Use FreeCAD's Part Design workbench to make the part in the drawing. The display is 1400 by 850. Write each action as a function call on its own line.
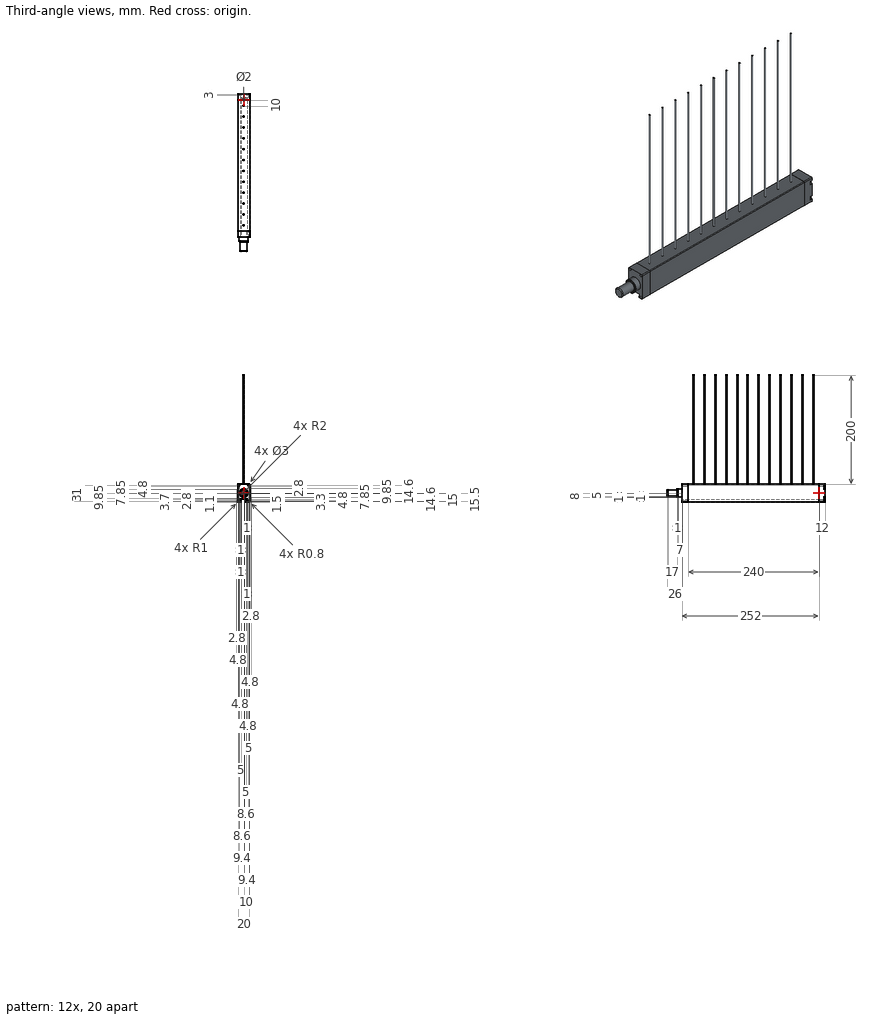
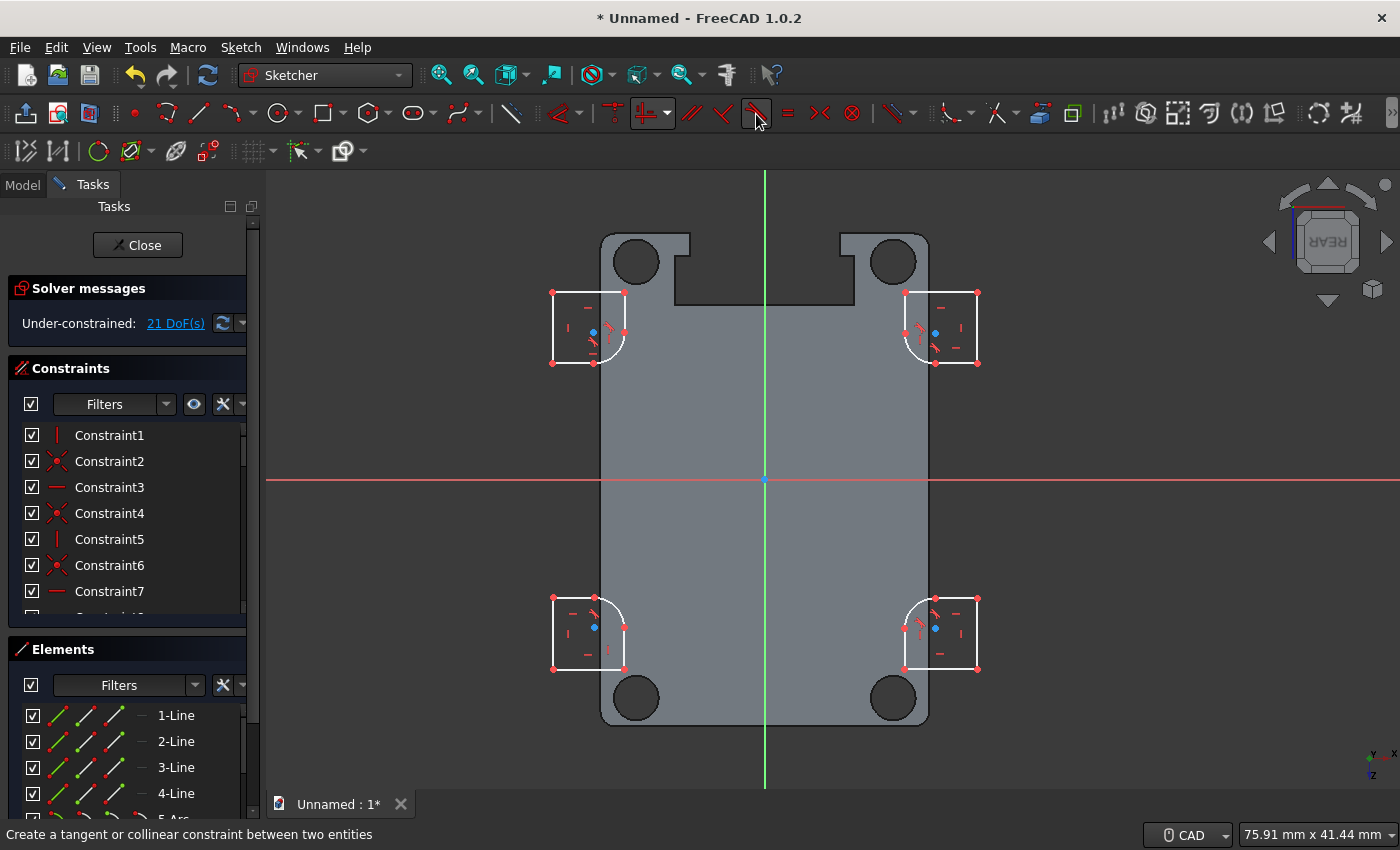
click(624, 657)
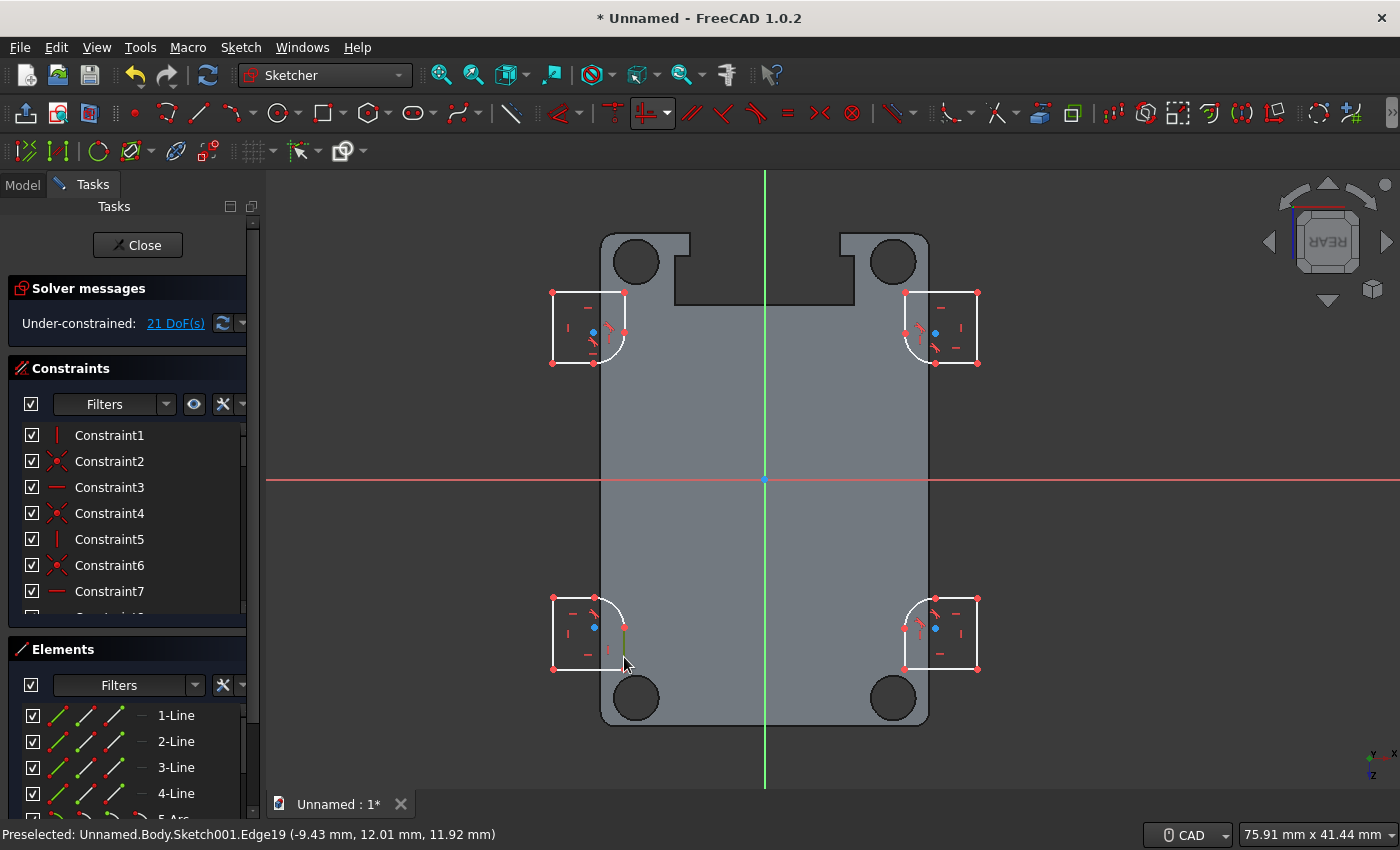
click(621, 614)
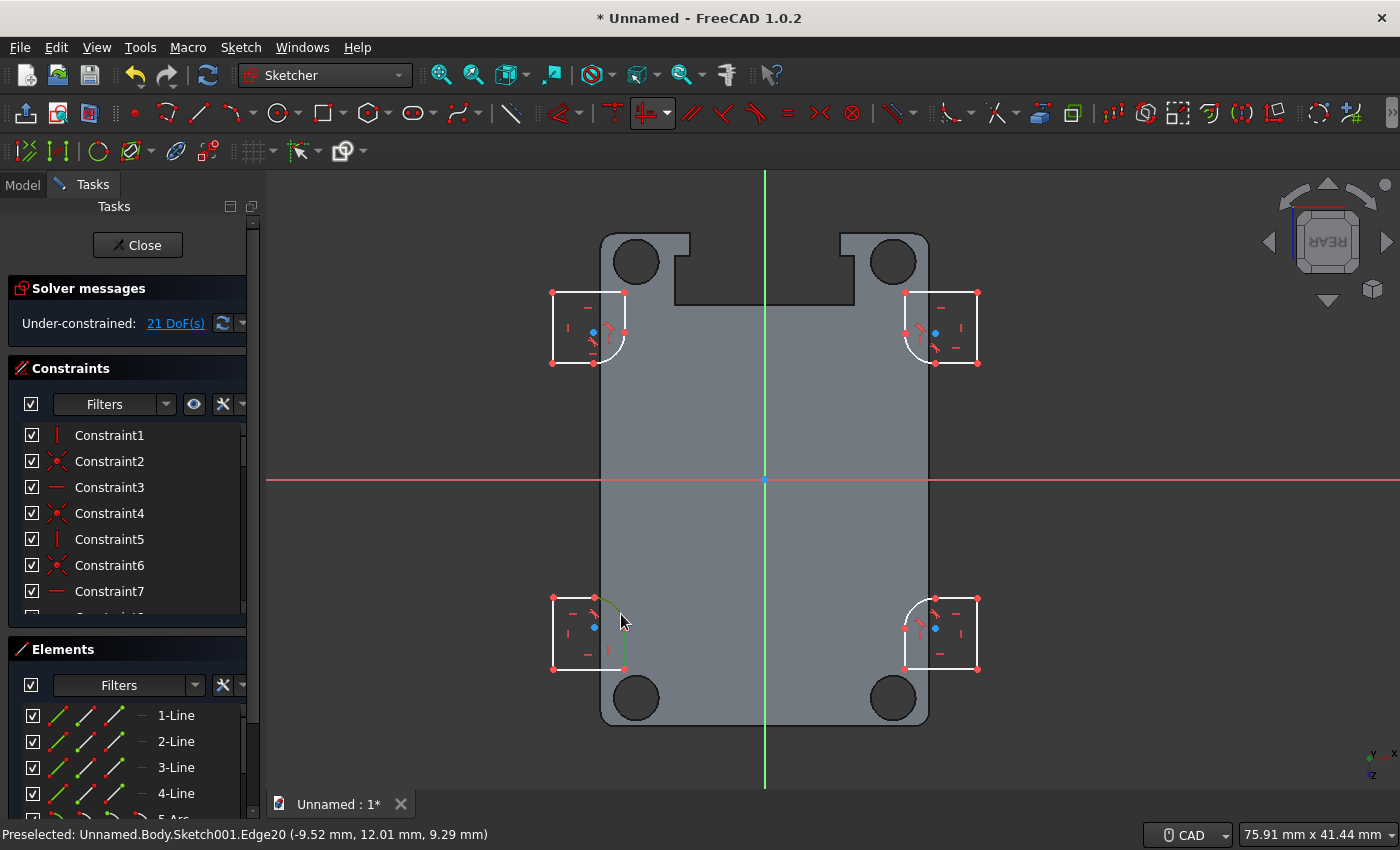
click(756, 114)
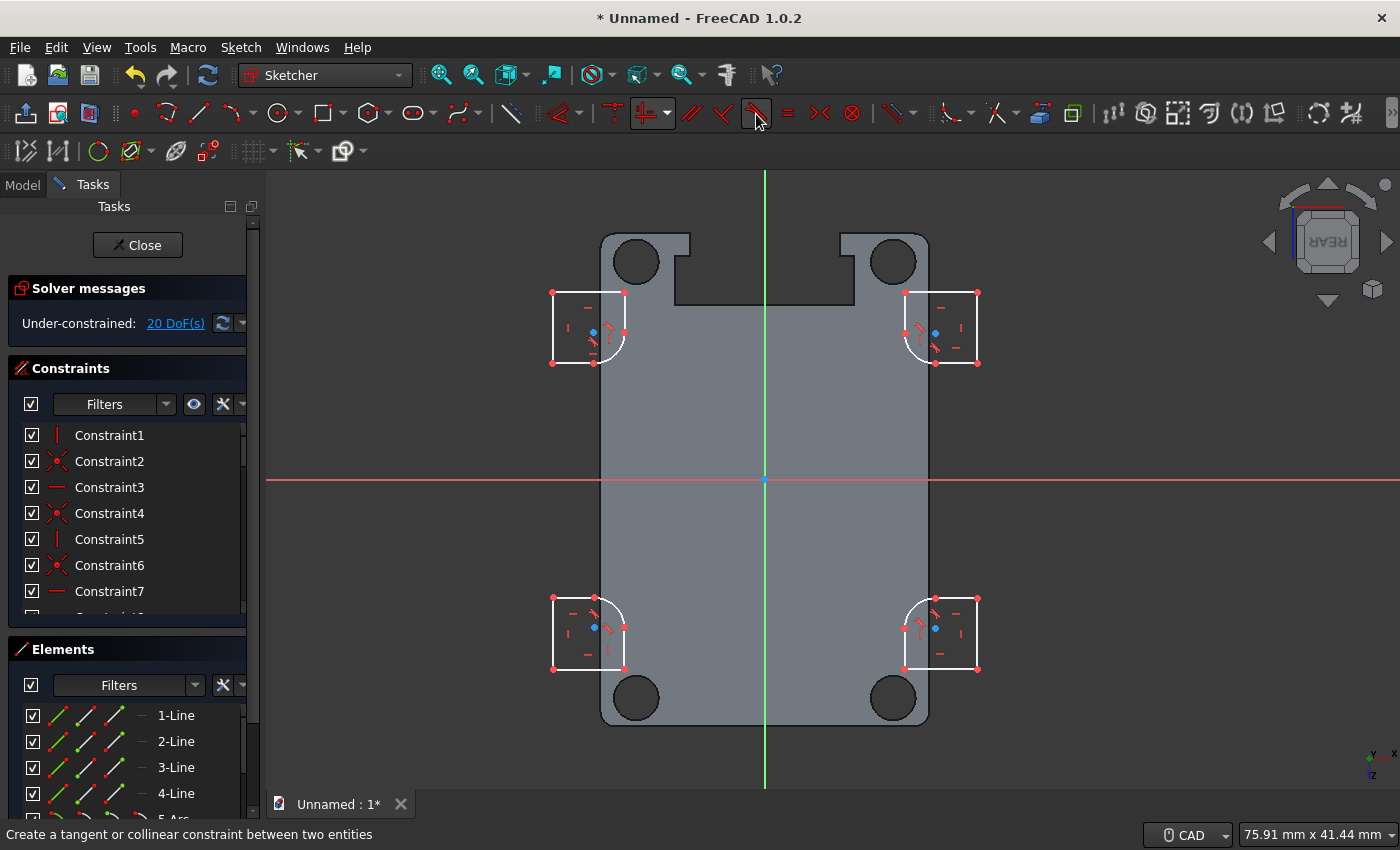
click(608, 360)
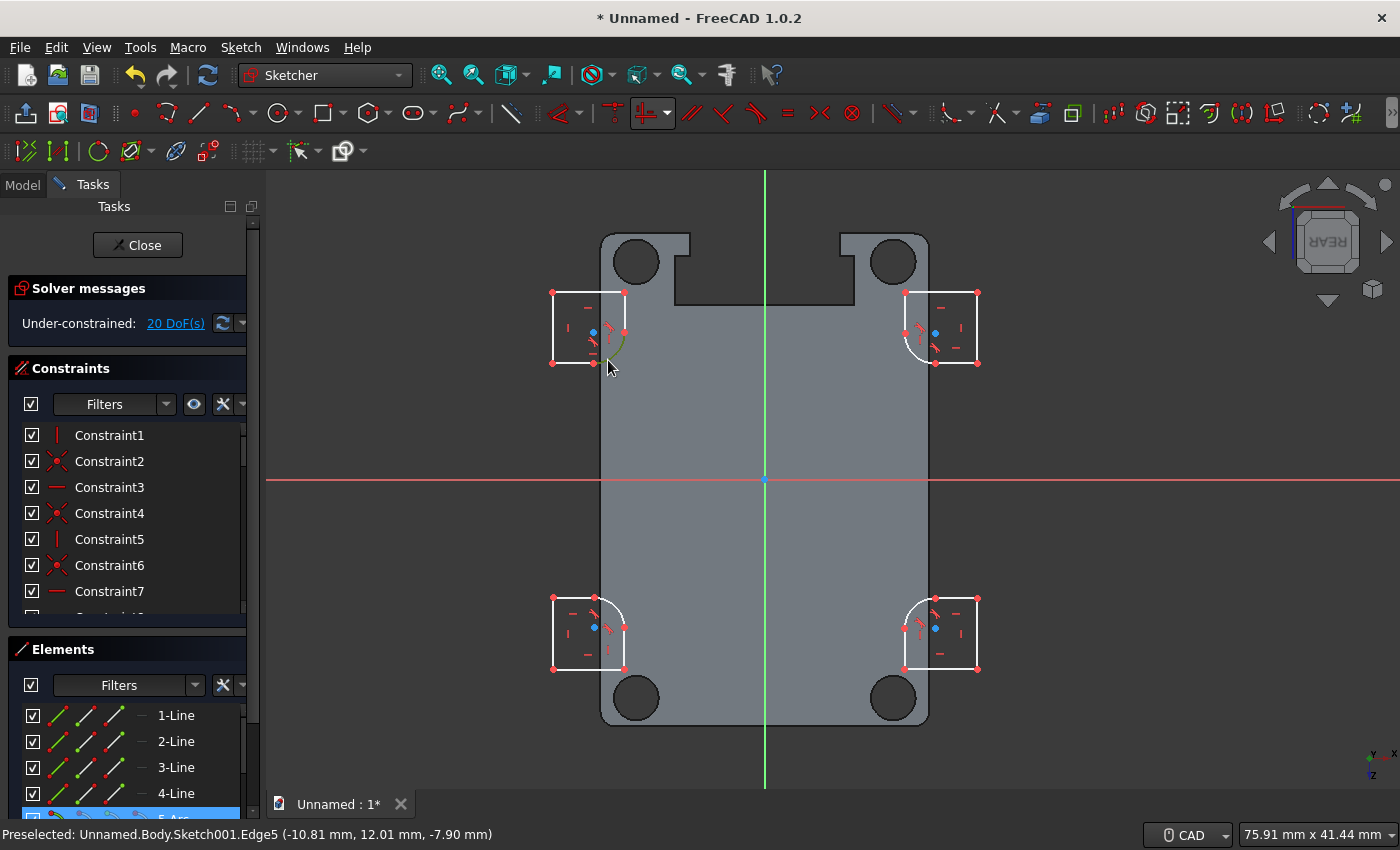
click(908, 347)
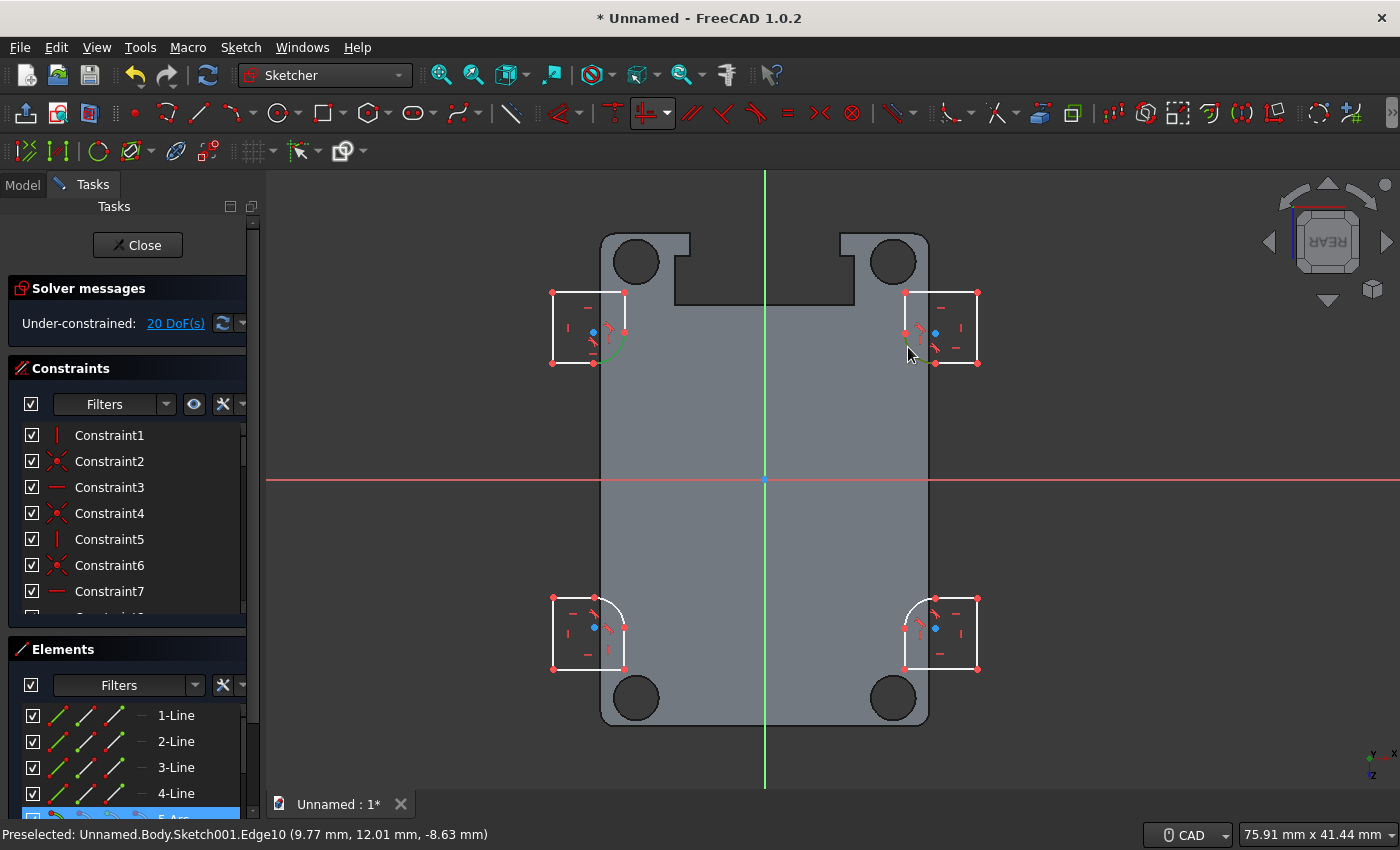
click(921, 602)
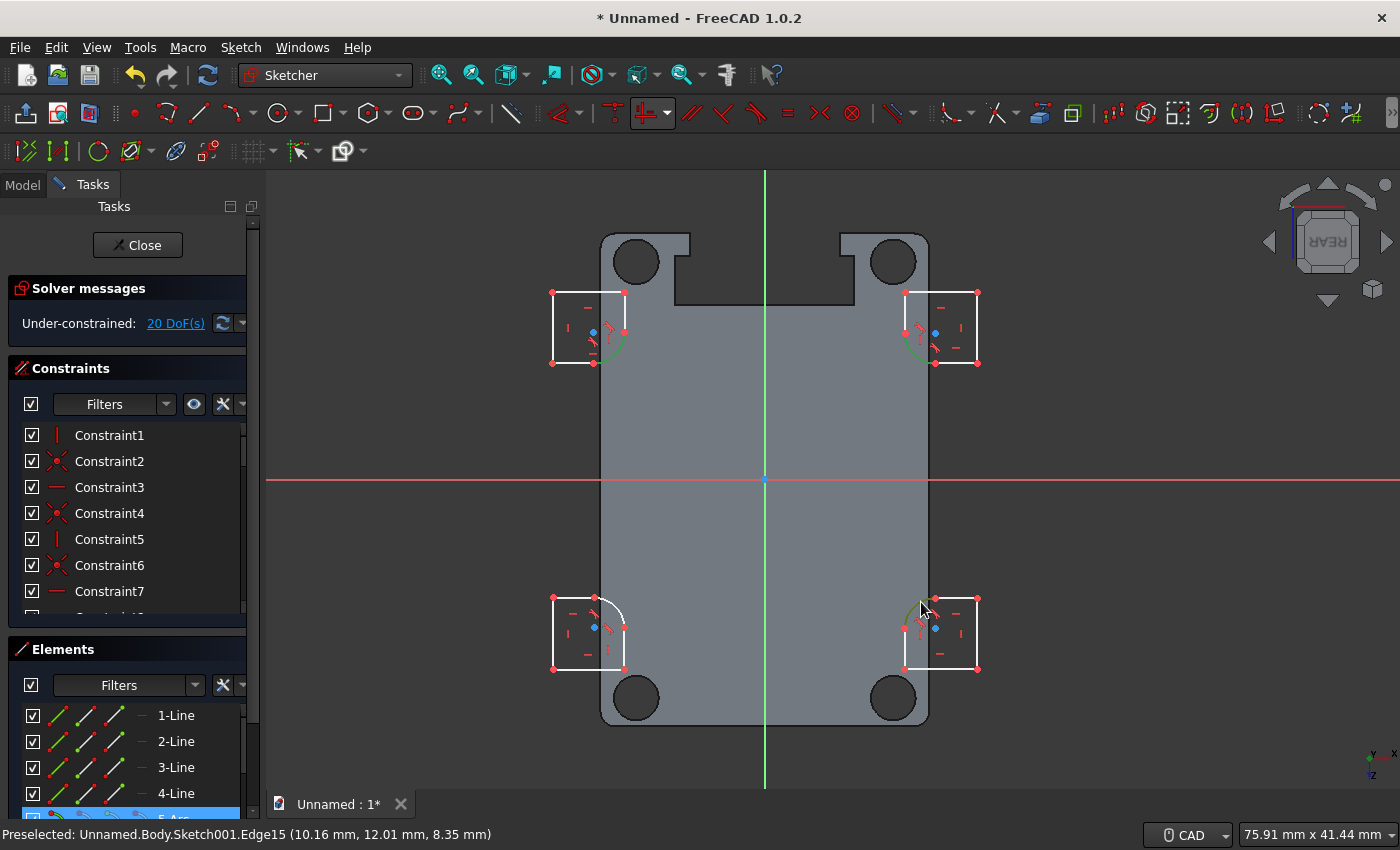
click(621, 614)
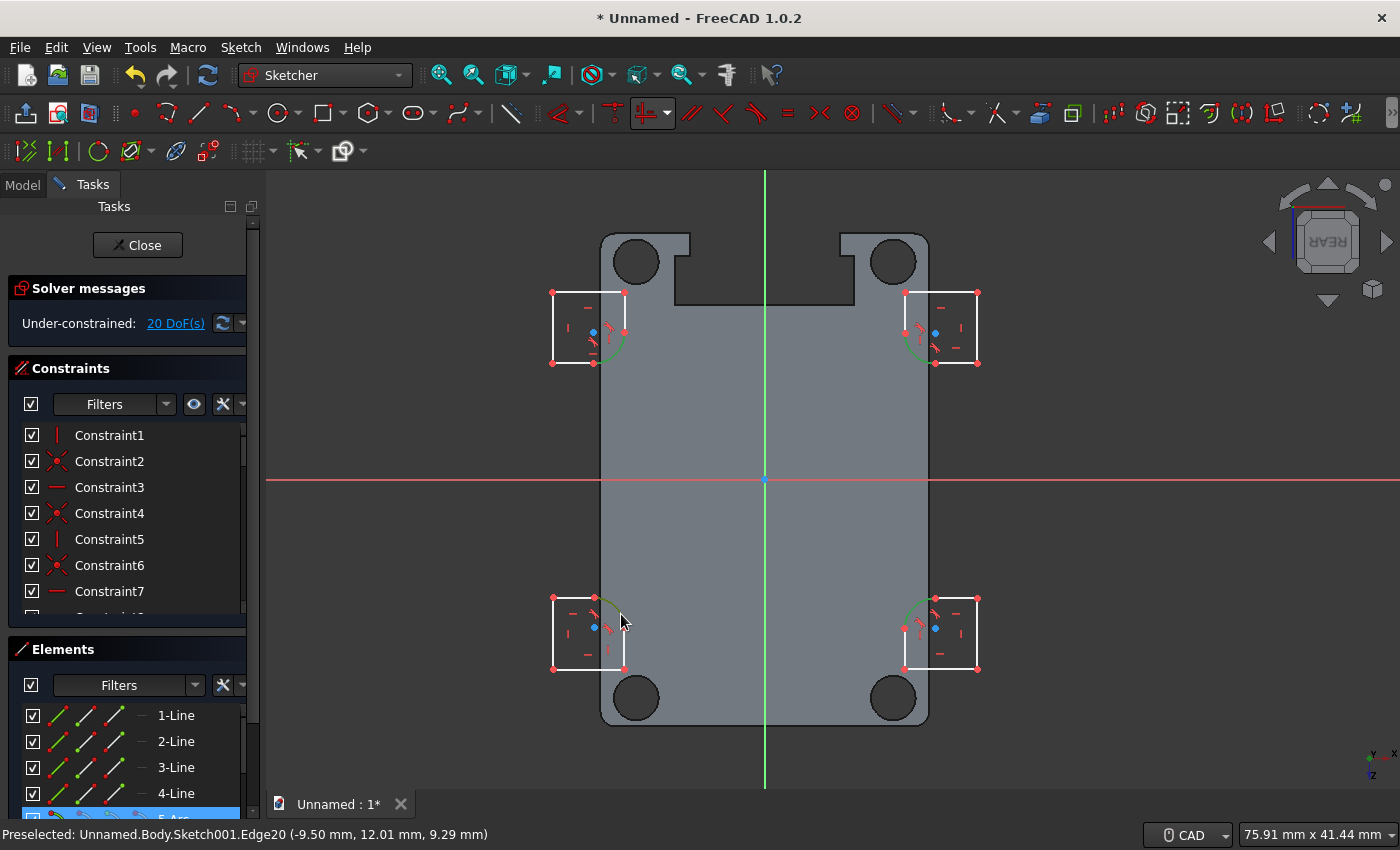
click(788, 114)